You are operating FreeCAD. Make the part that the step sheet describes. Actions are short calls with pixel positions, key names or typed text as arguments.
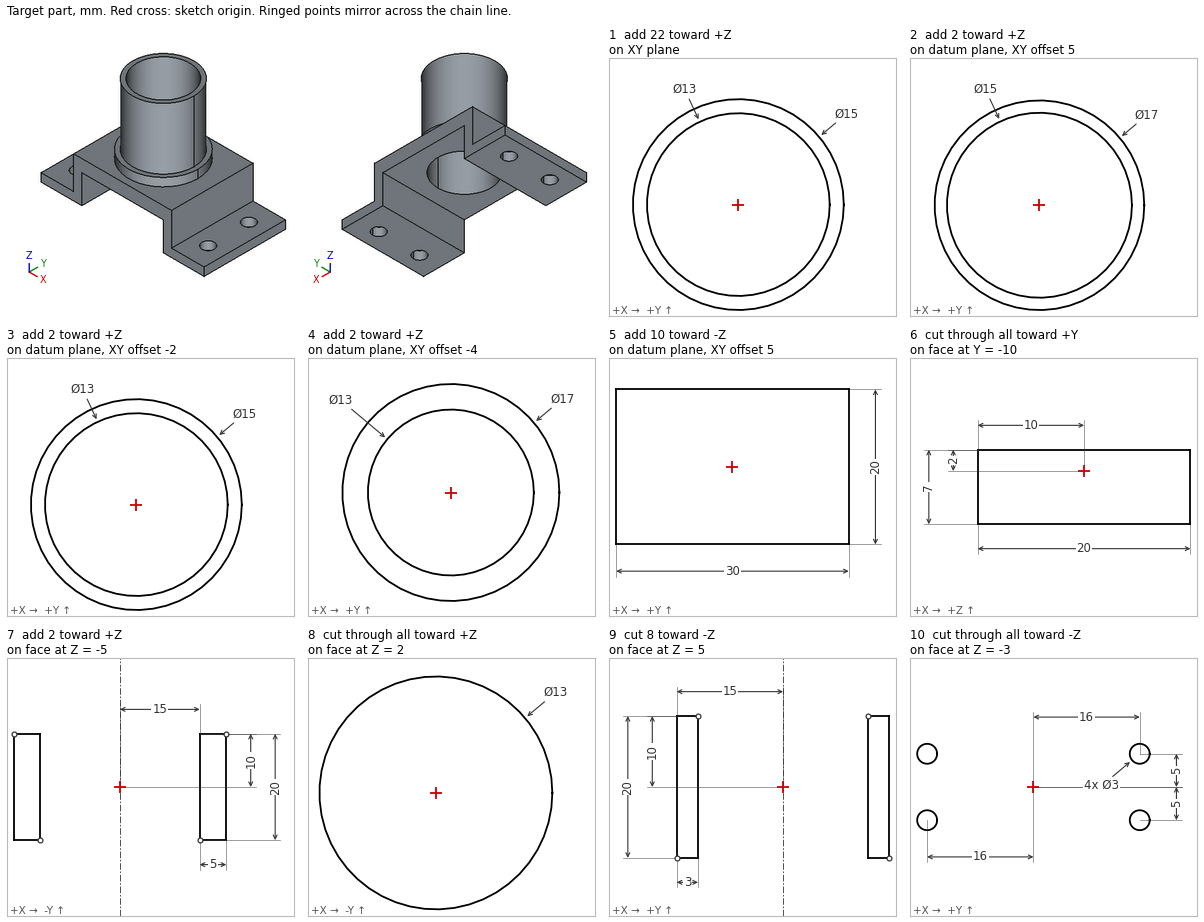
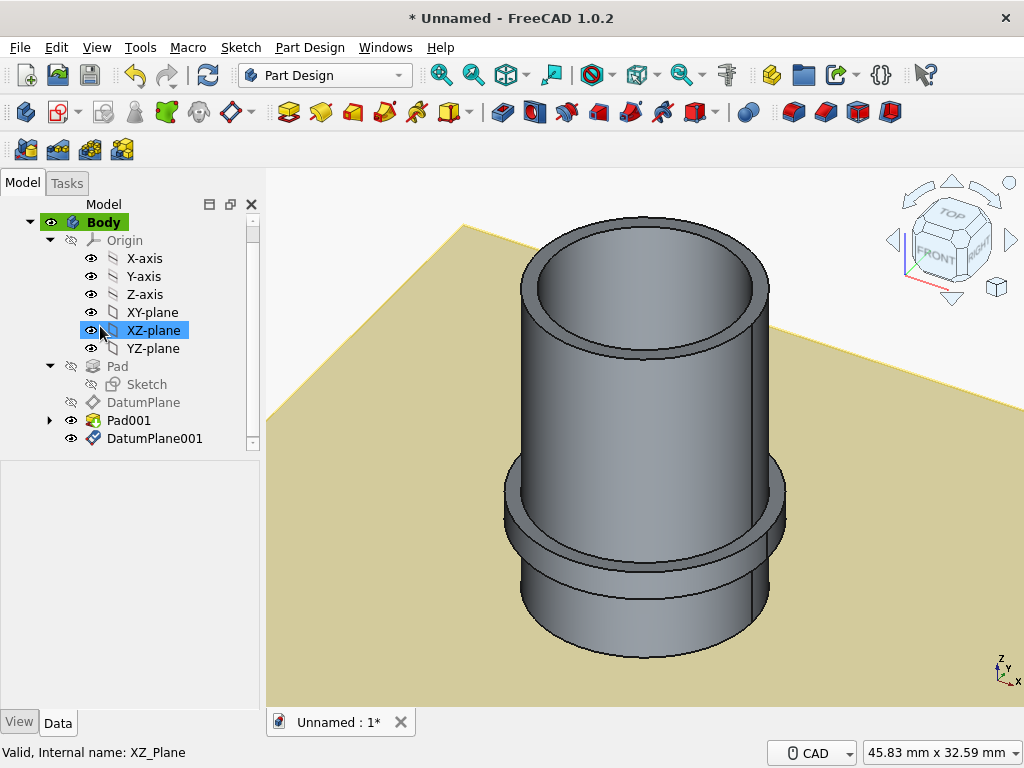
click(116, 438)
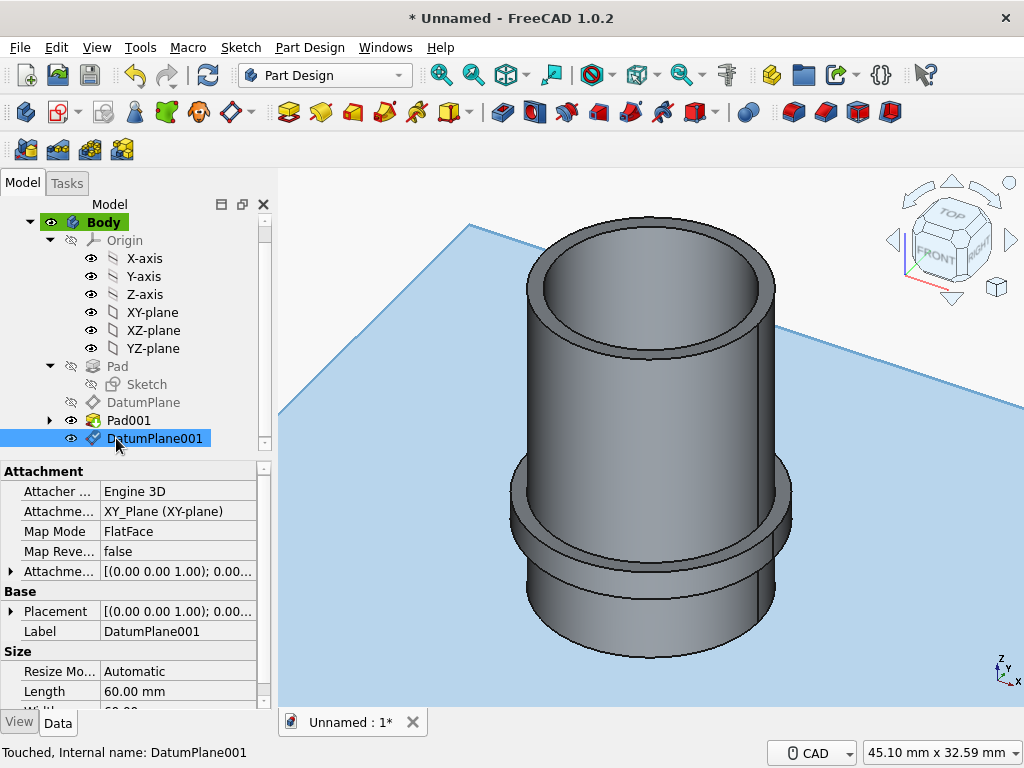
click(58, 112)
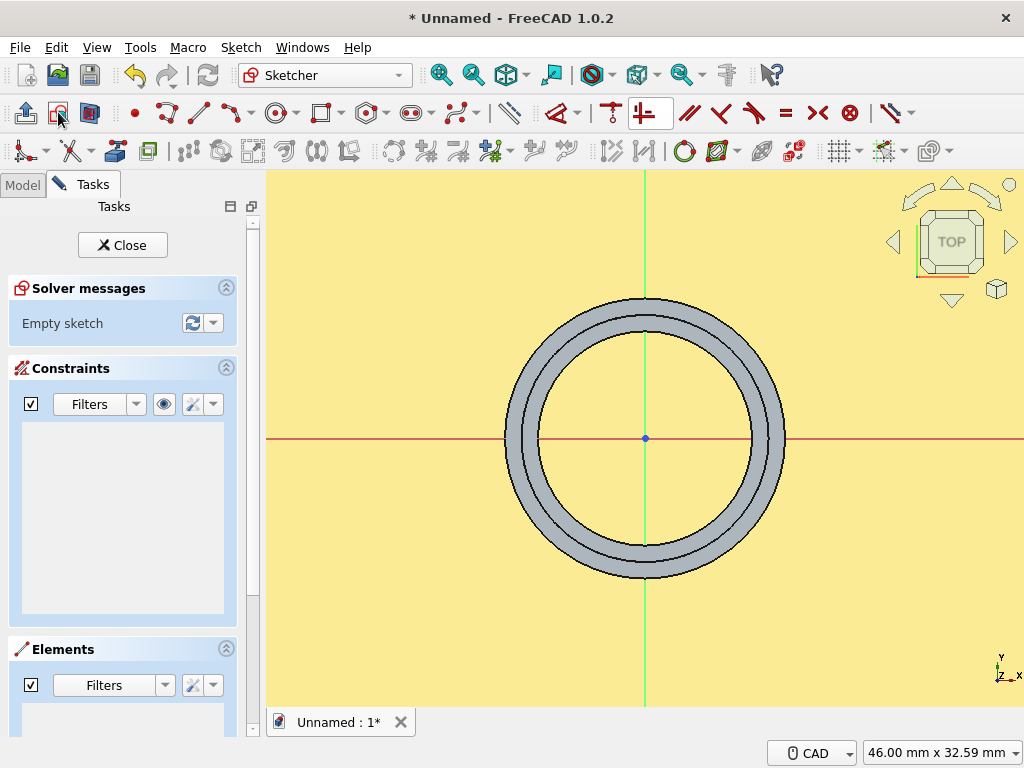
click(90, 114)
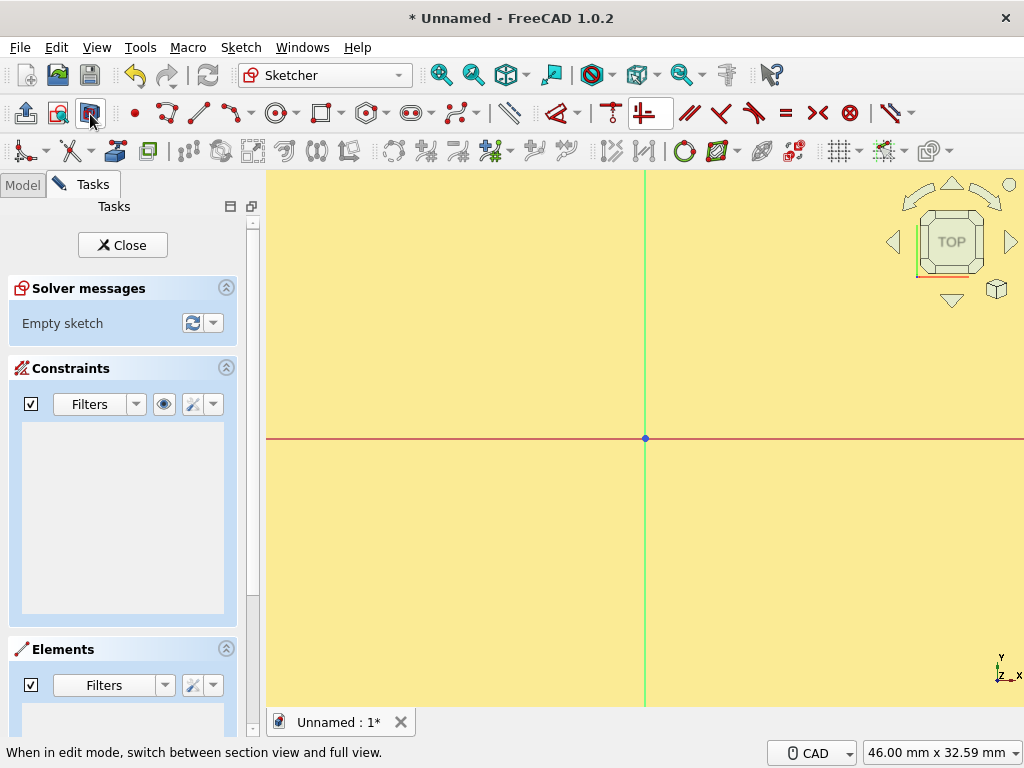
scroll(784, 439, up, 2)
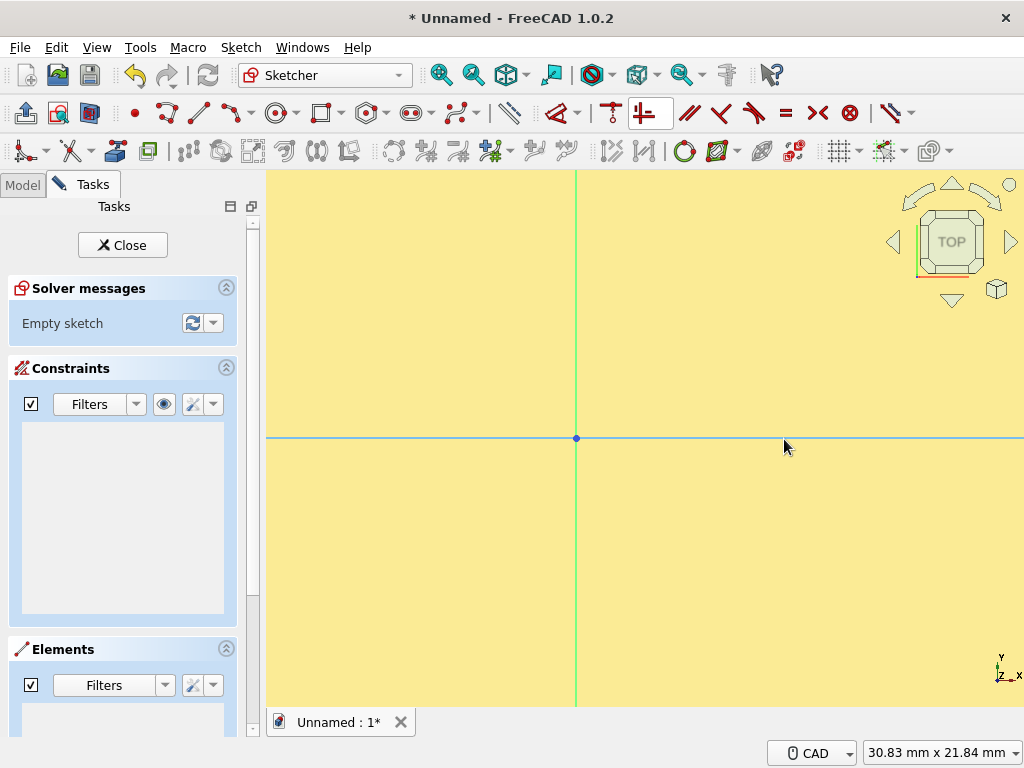
click(276, 114)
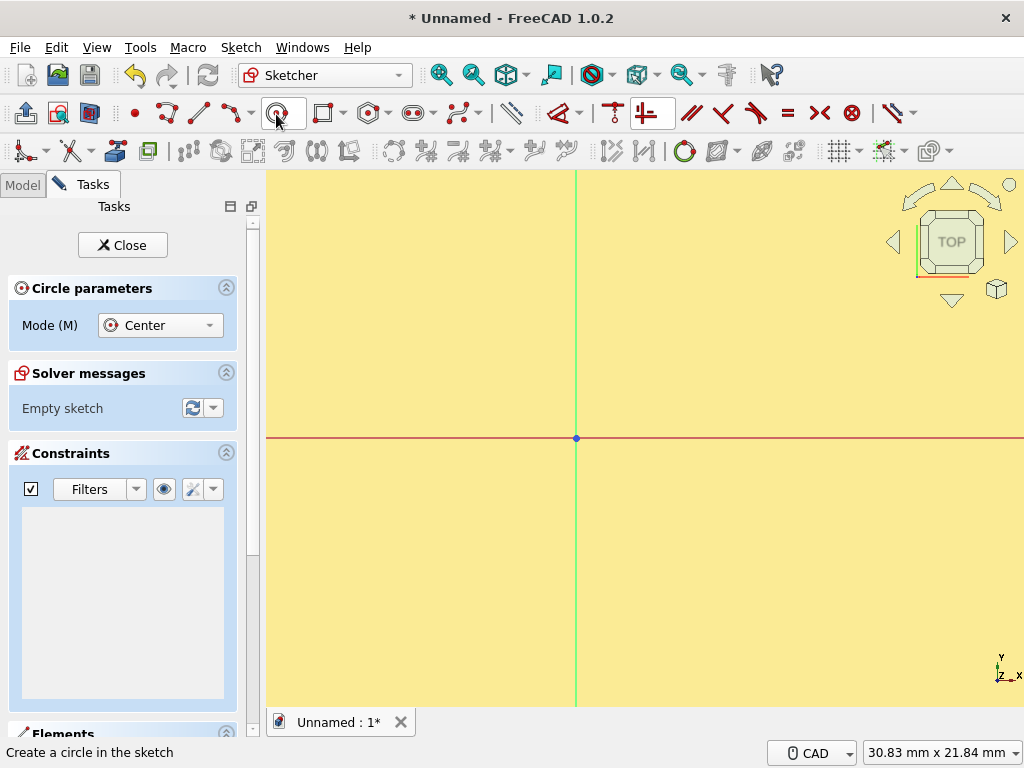
click(576, 438)
click(707, 308)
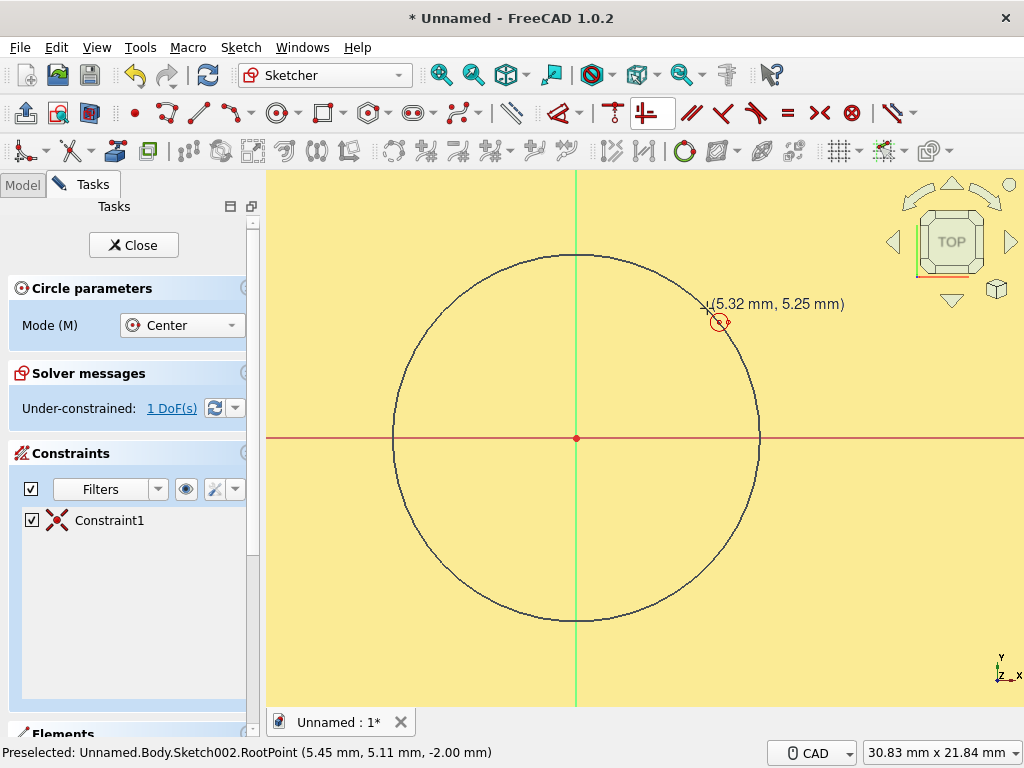
click(576, 438)
click(689, 325)
key(Escape)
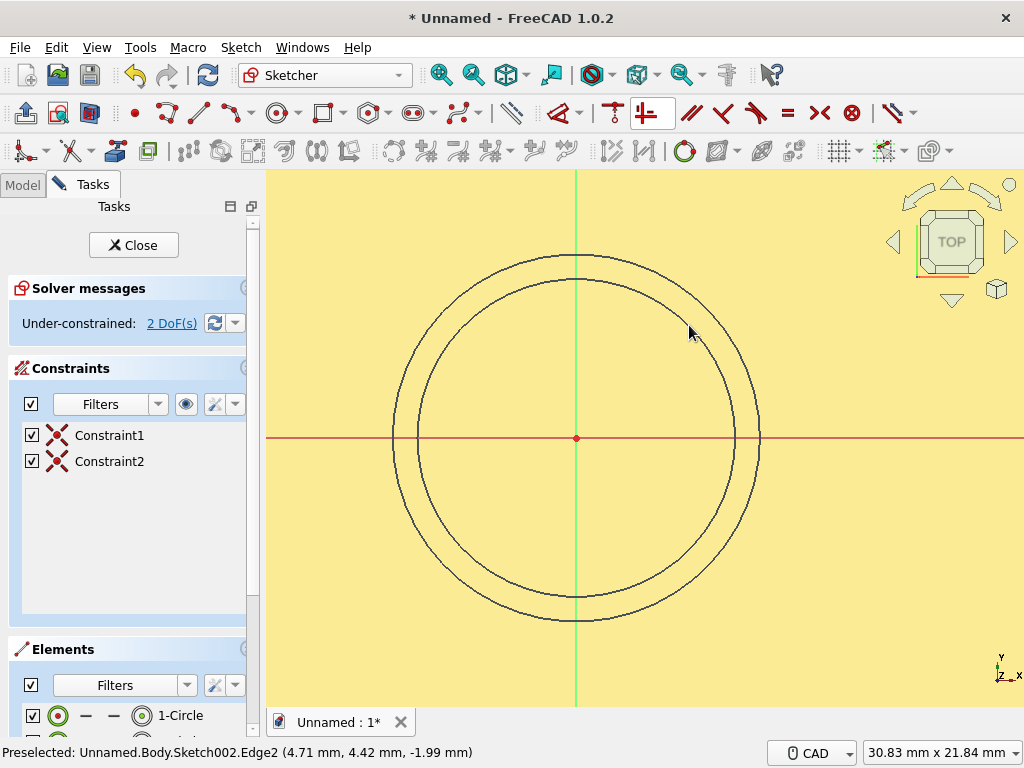
key(d)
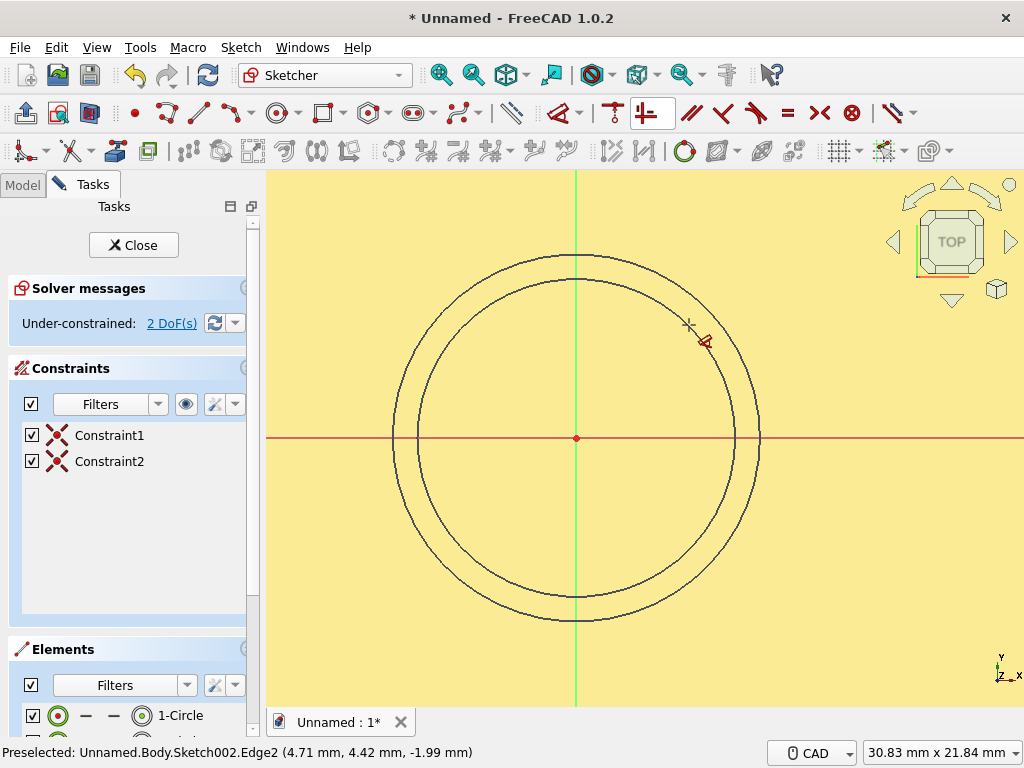
click(706, 308)
click(729, 285)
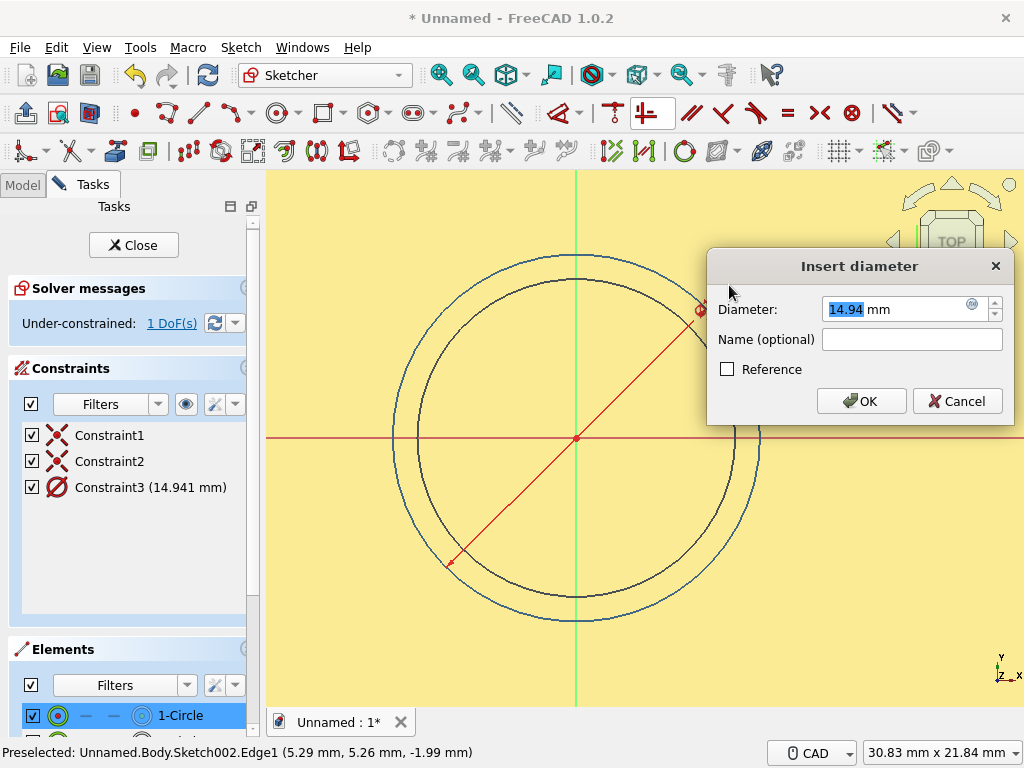
text(15)
key(Return)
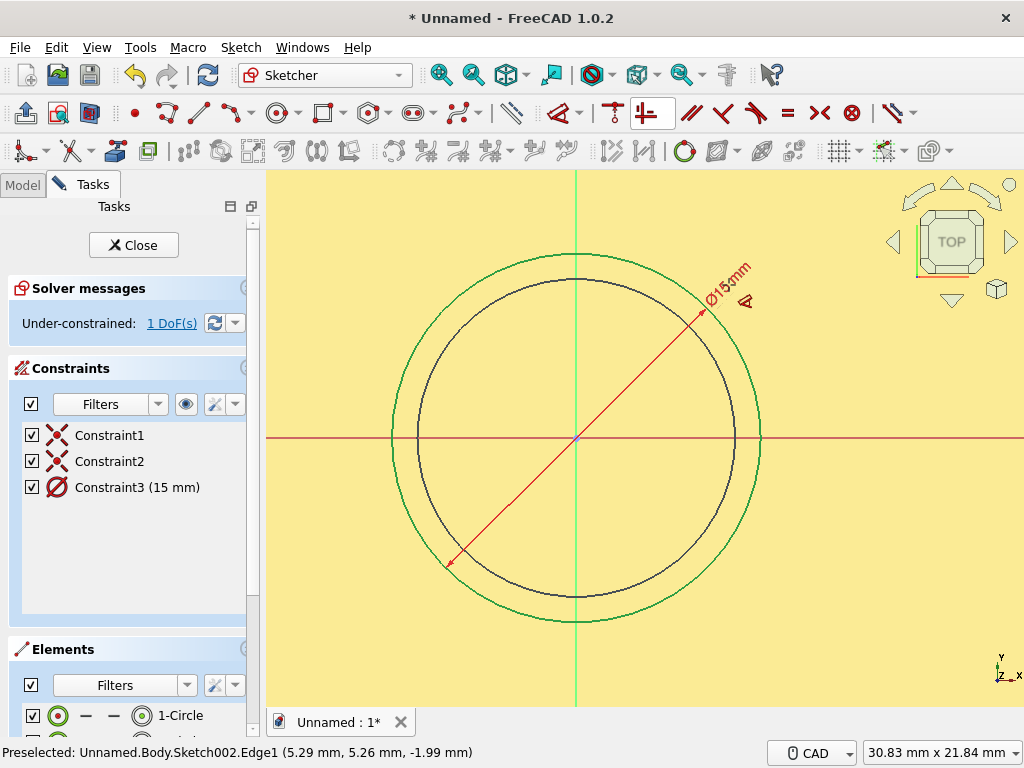
click(688, 325)
click(781, 377)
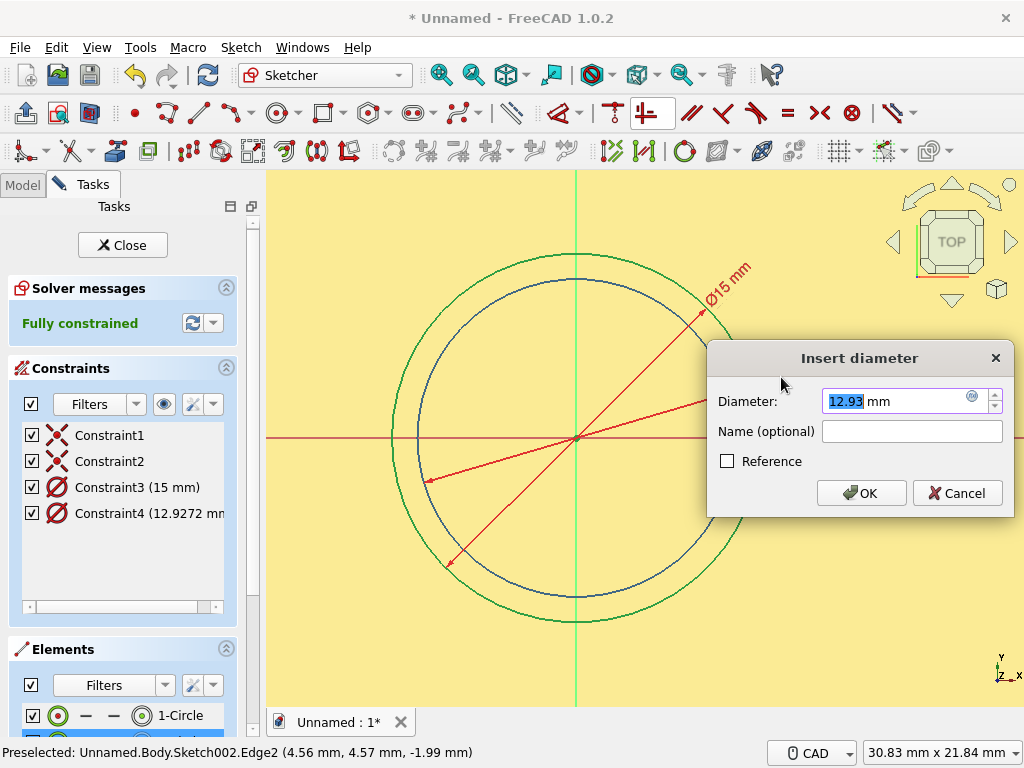
text(13)
key(Return)
key(Escape)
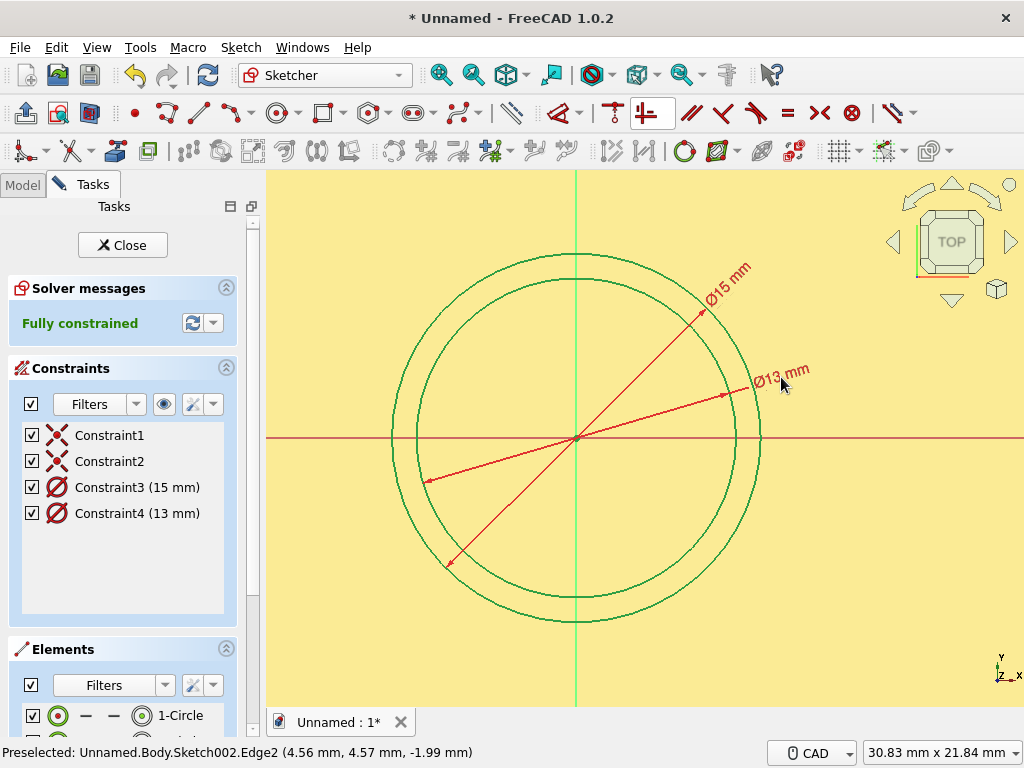
click(123, 245)